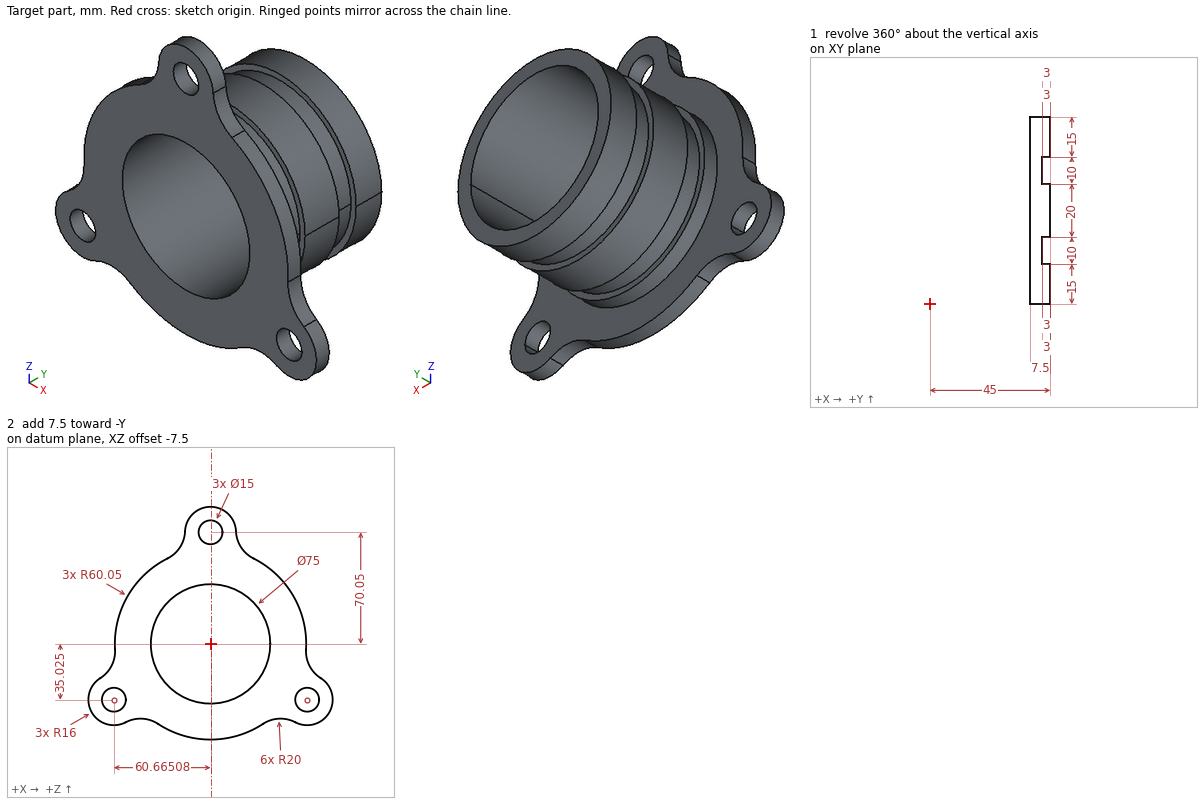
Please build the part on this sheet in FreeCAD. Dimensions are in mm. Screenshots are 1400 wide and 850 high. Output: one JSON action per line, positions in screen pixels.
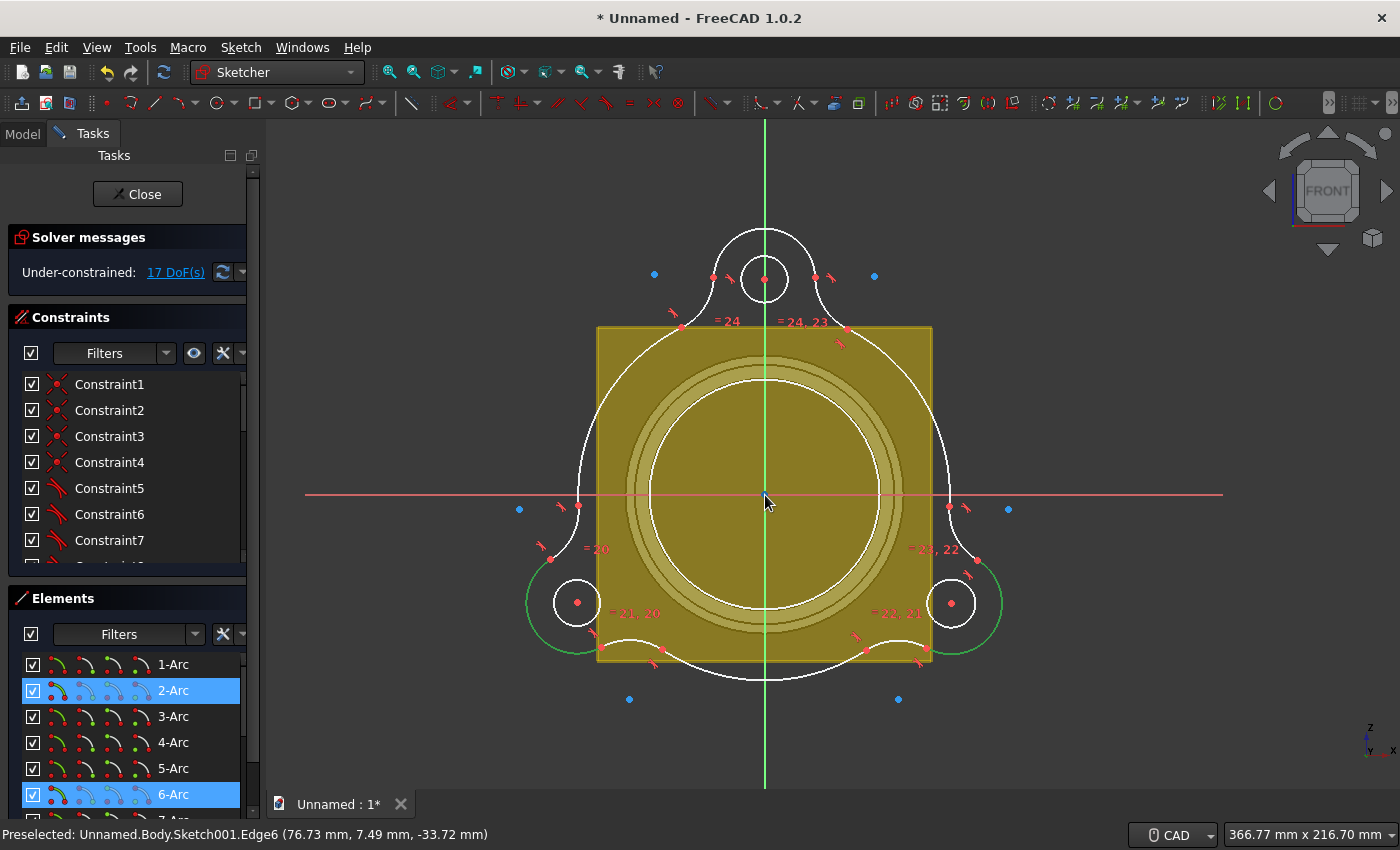
{"action": "left_click", "coordinate": [794, 238]}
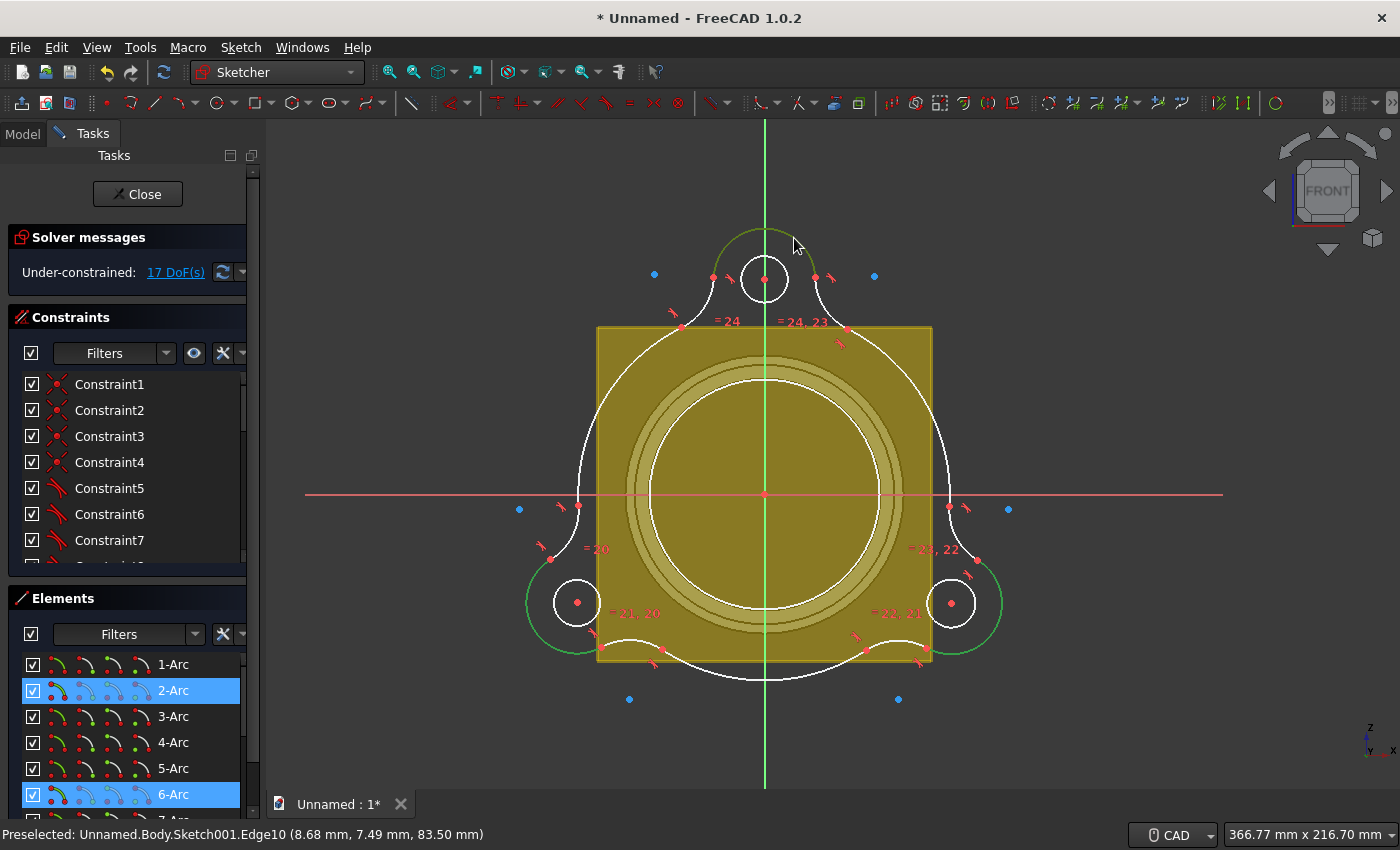
{"action": "left_click", "coordinate": [630, 104]}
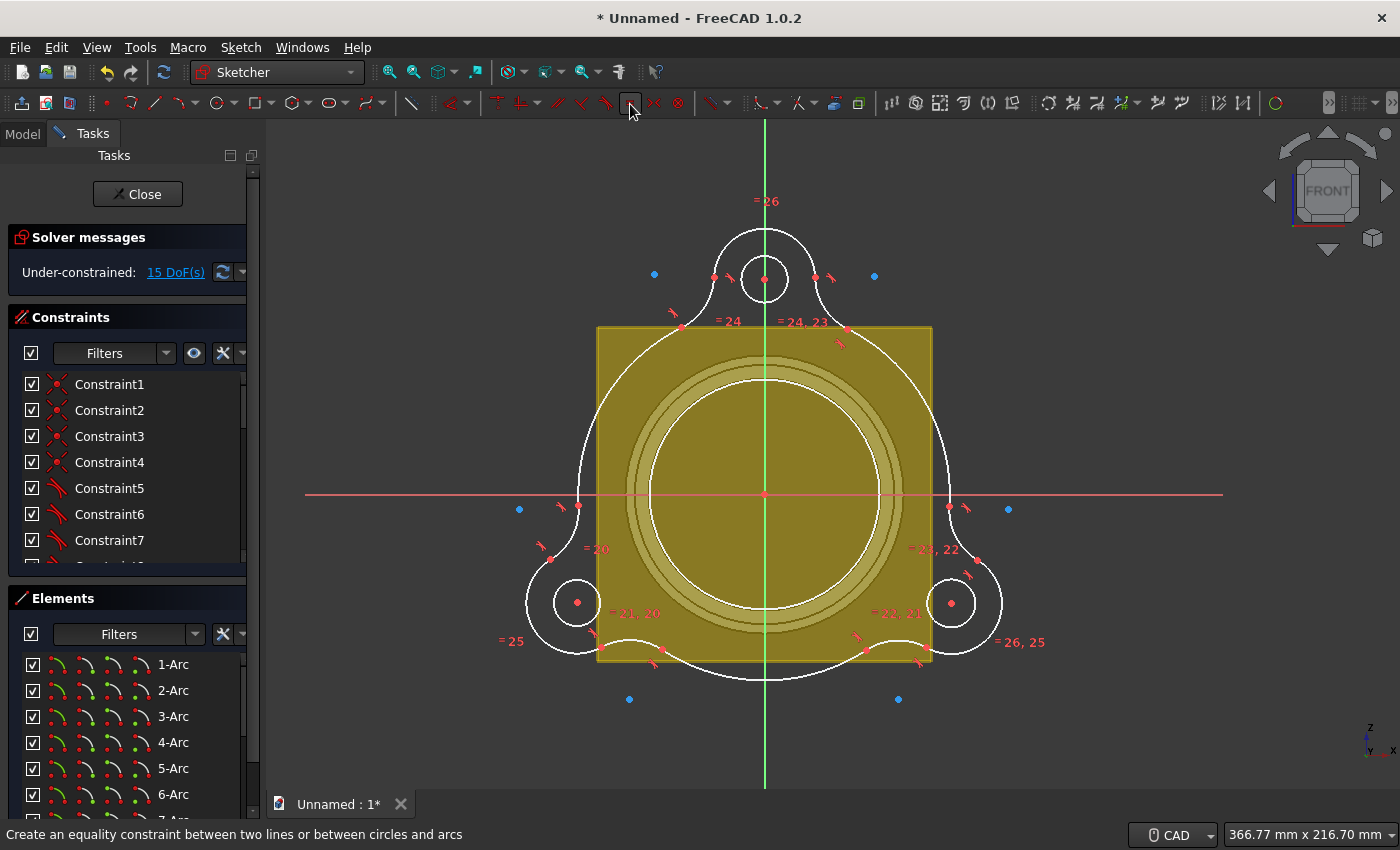
{"action": "left_click", "coordinate": [721, 675]}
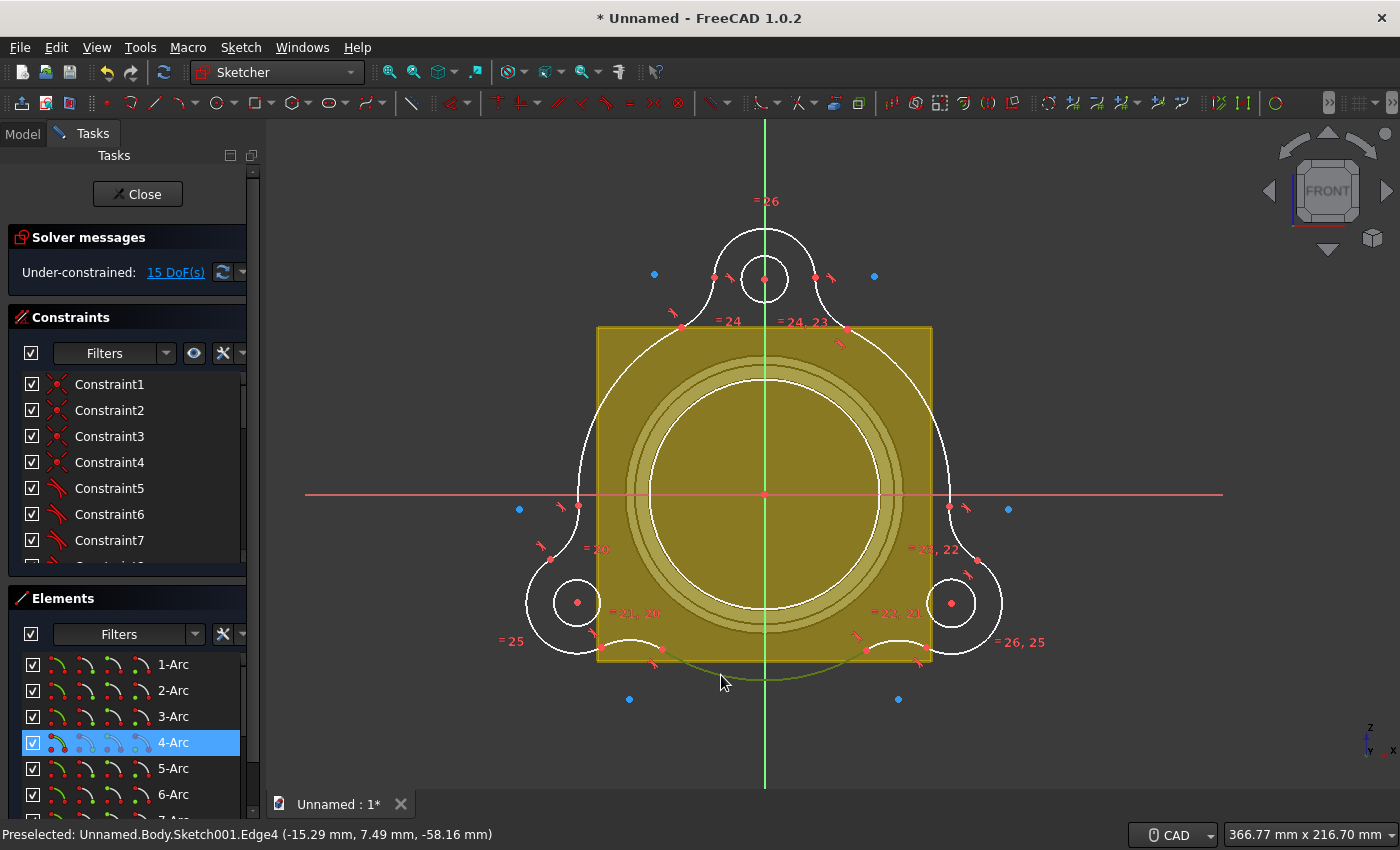
{"action": "left_click", "coordinate": [942, 442]}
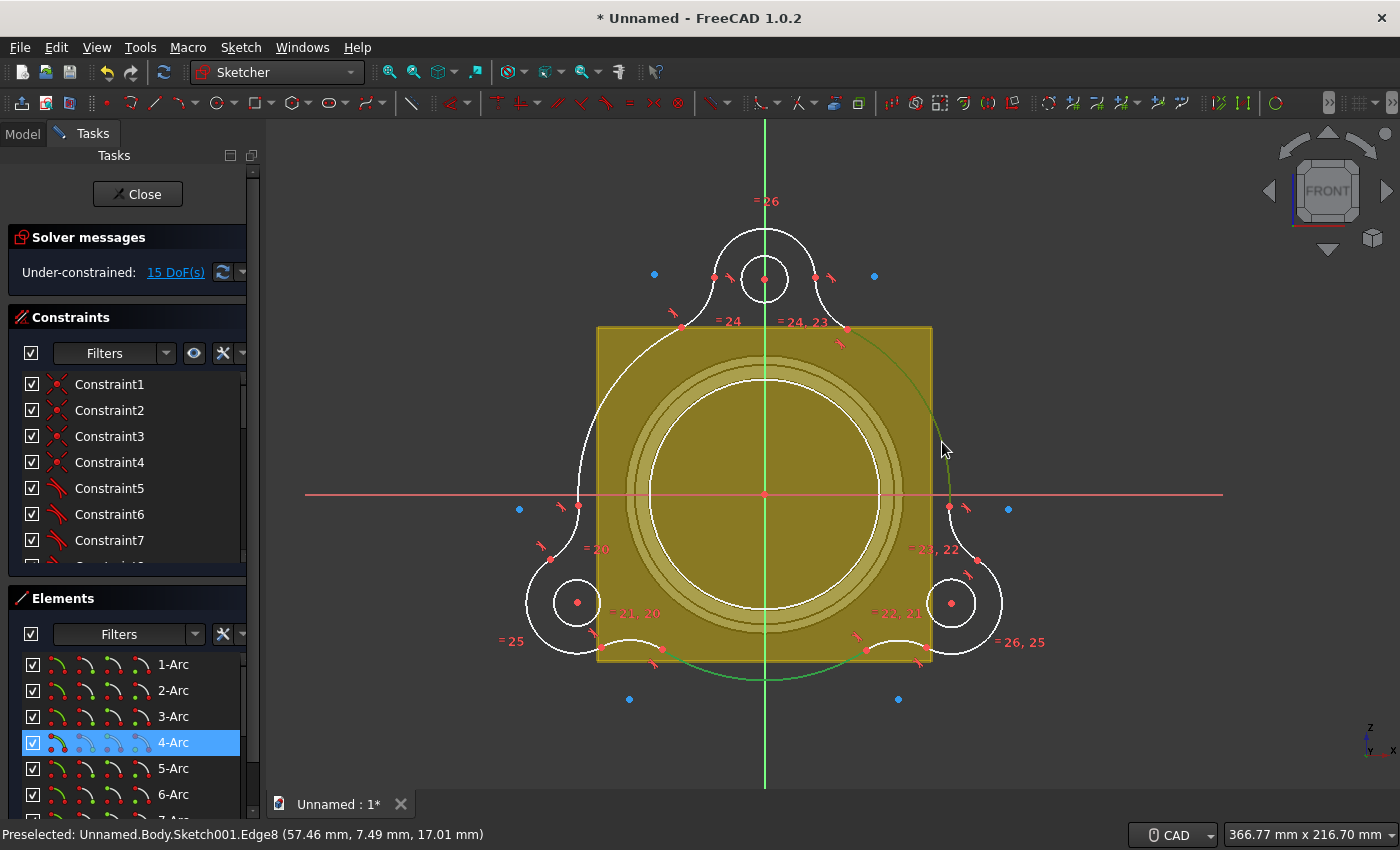
{"action": "left_click", "coordinate": [629, 367]}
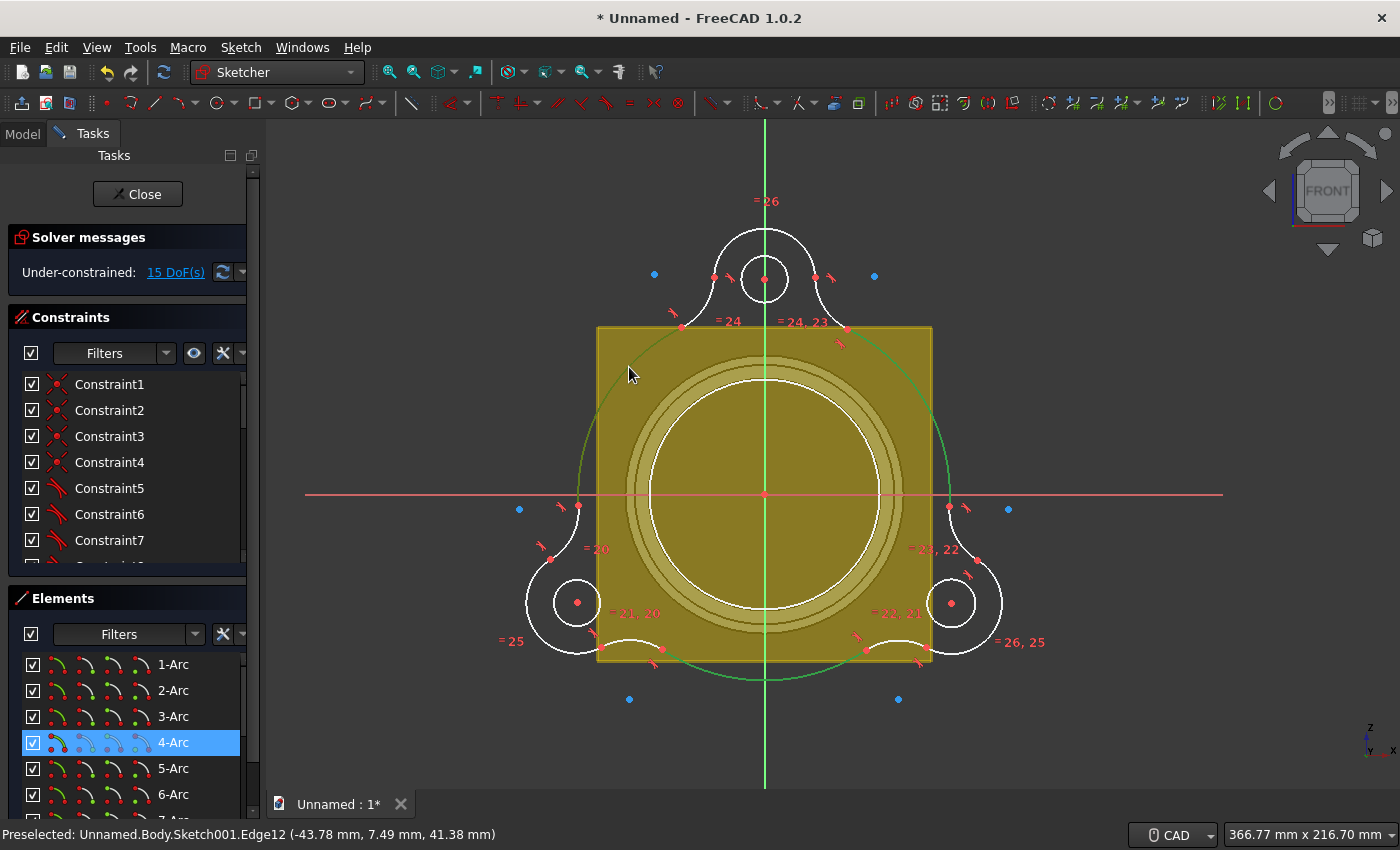
{"action": "key", "text": "e"}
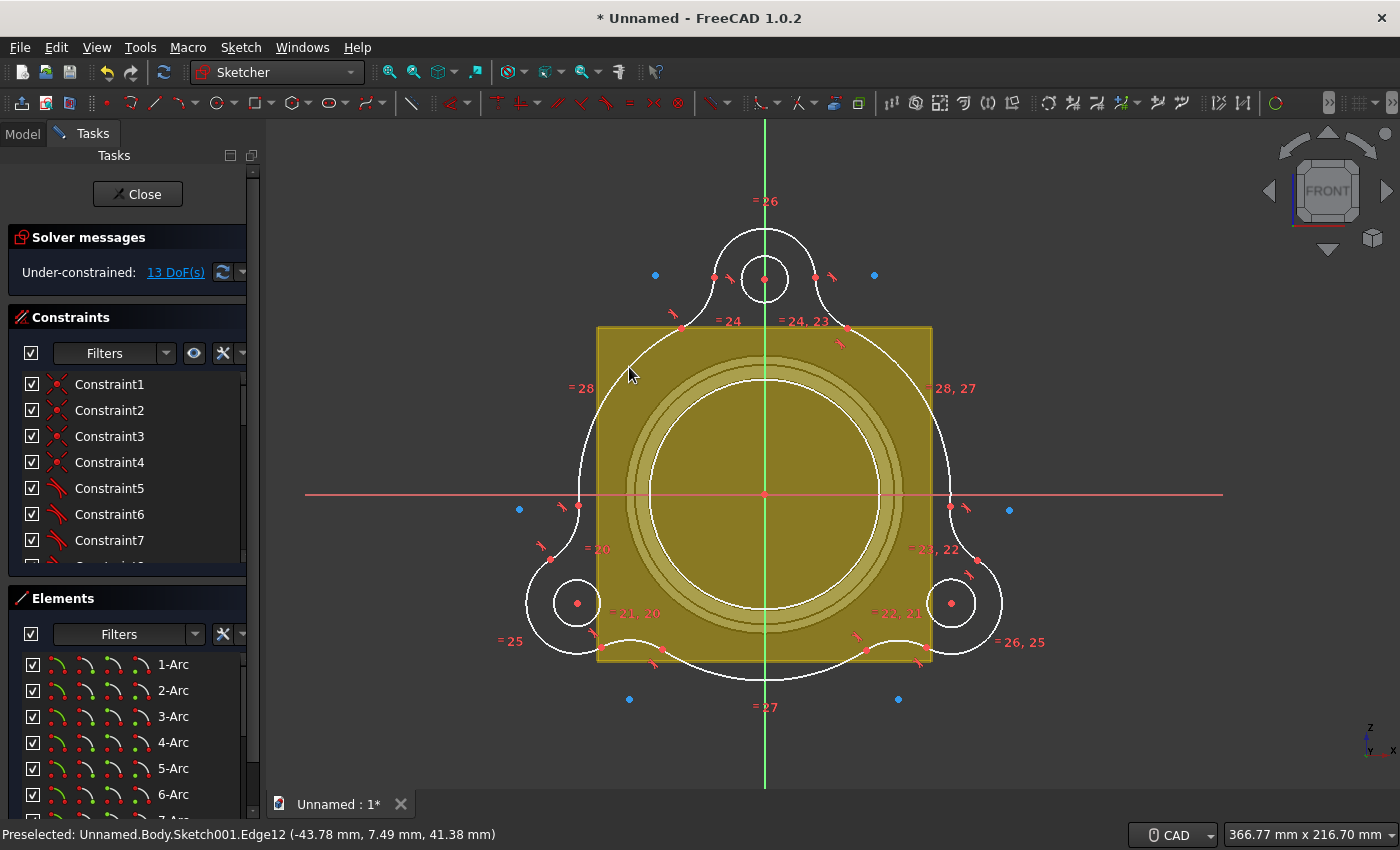
{"action": "left_click", "coordinate": [593, 587]}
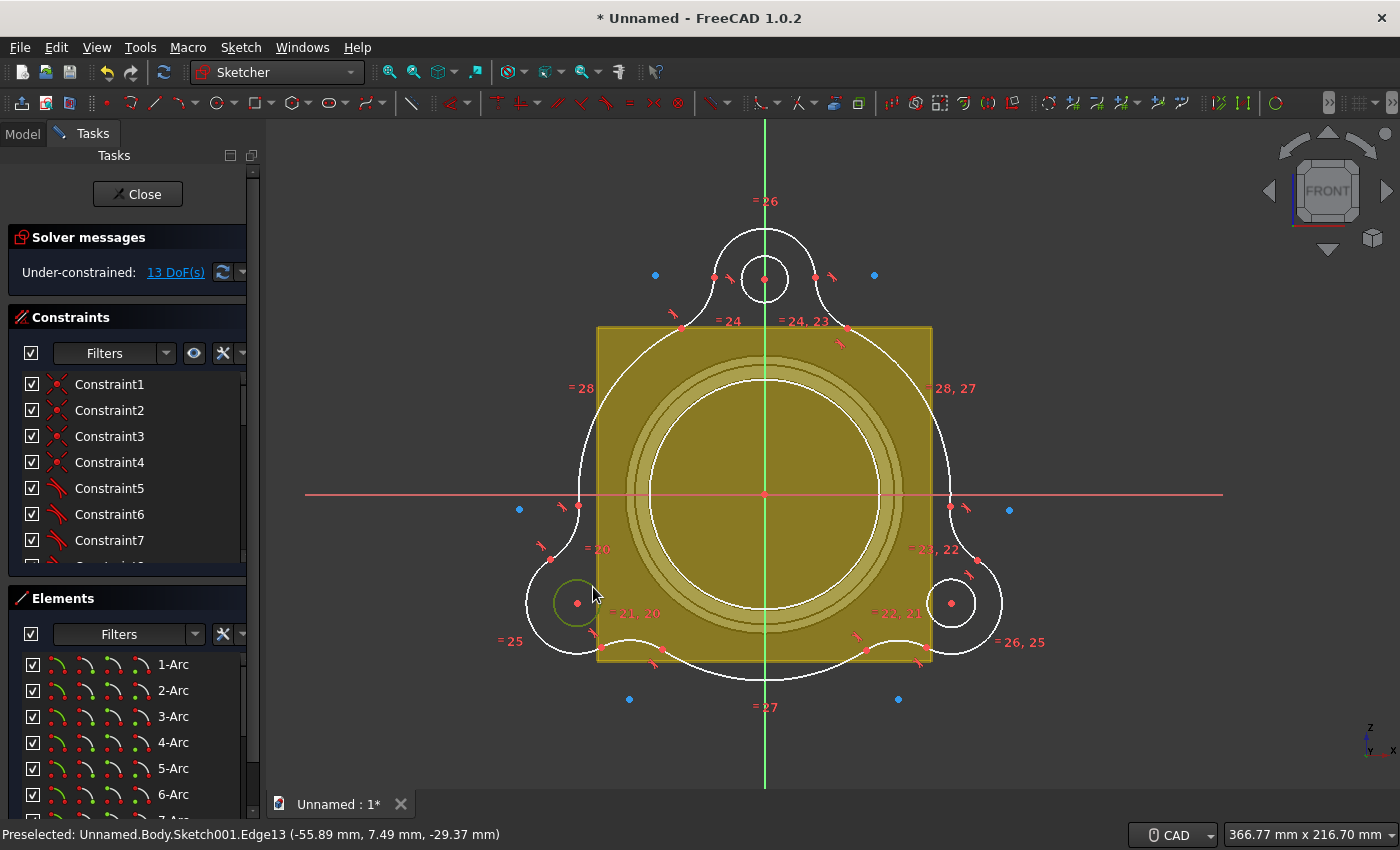
{"action": "left_click", "coordinate": [968, 586]}